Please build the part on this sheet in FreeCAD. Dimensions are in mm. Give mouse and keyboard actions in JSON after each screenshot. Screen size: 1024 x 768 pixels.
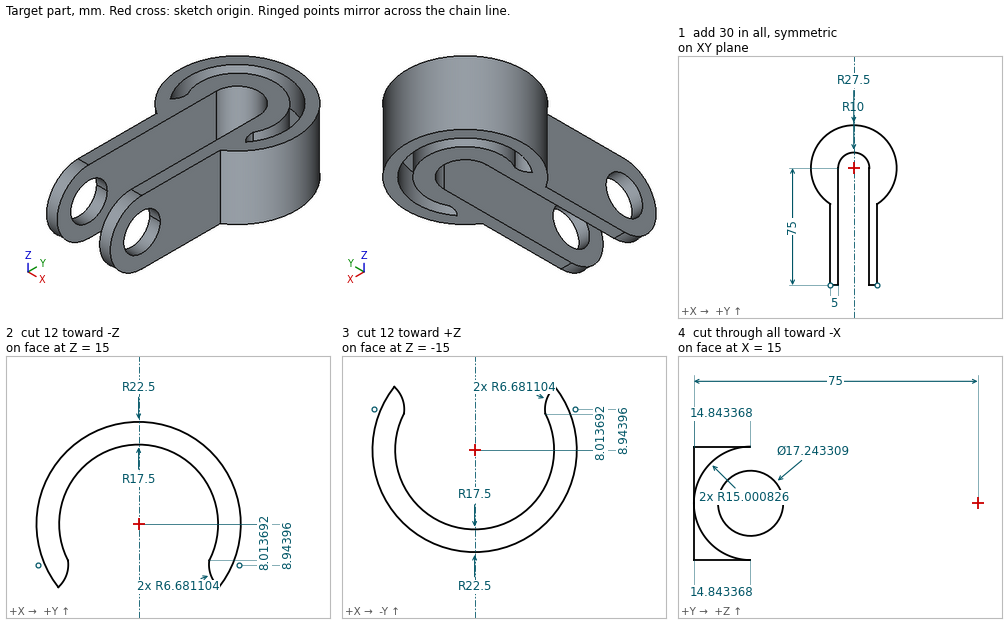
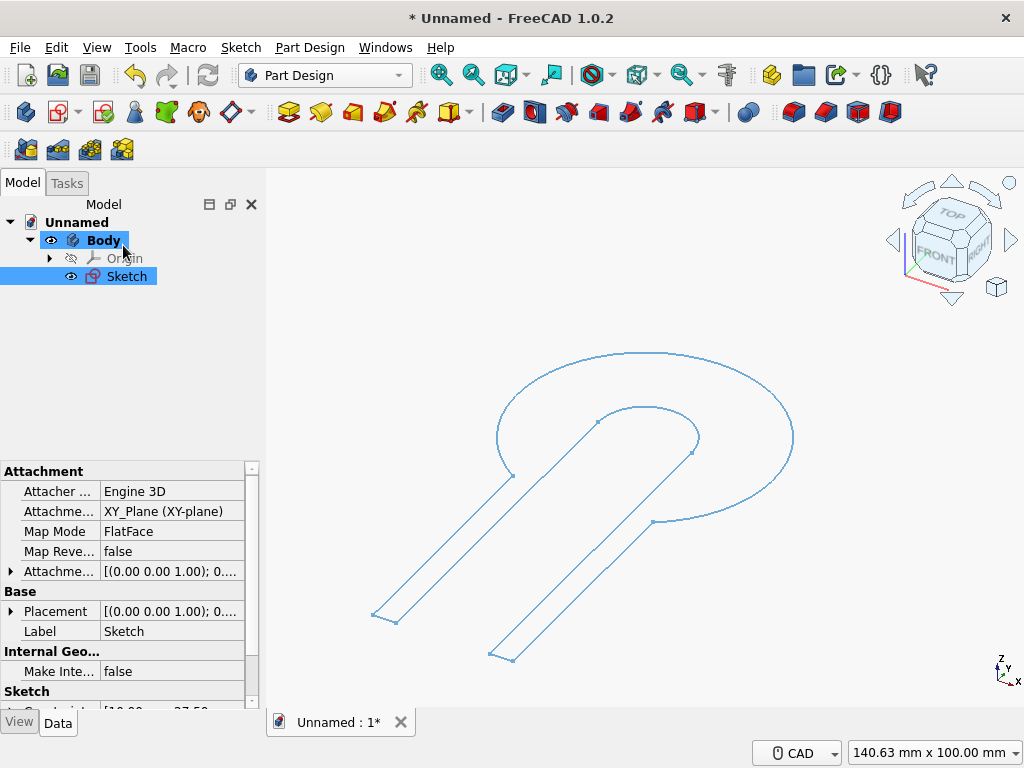
{"action": "left_click", "coordinate": [290, 112]}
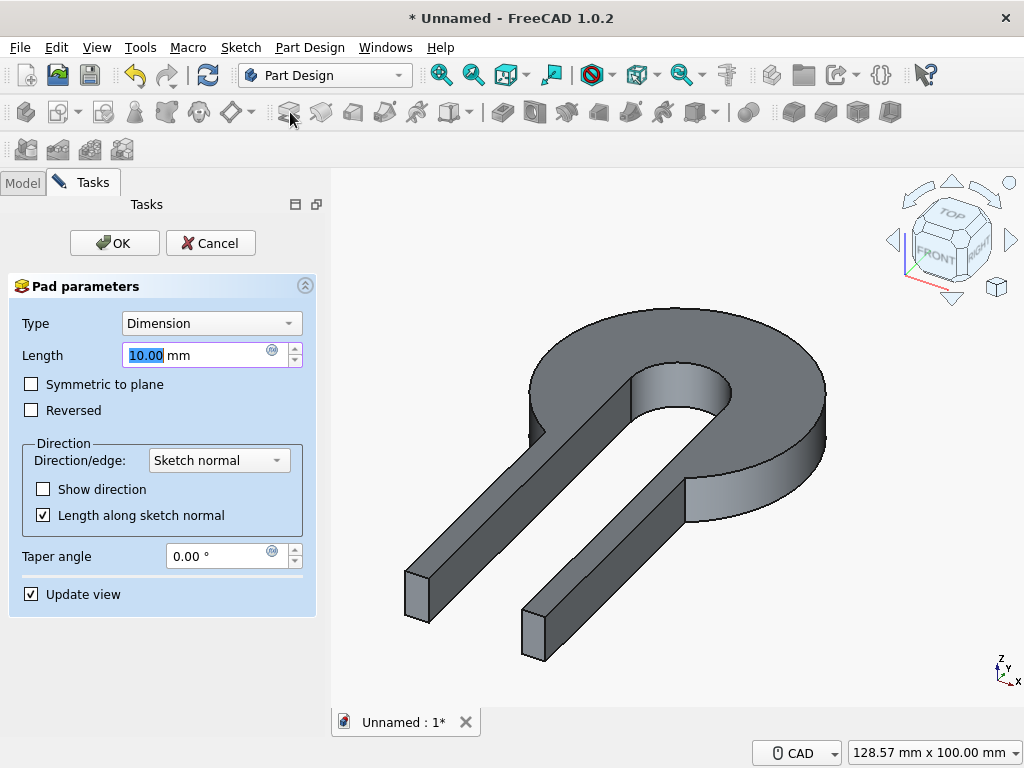
{"action": "type", "text": "30"}
{"action": "key", "text": "Tab"}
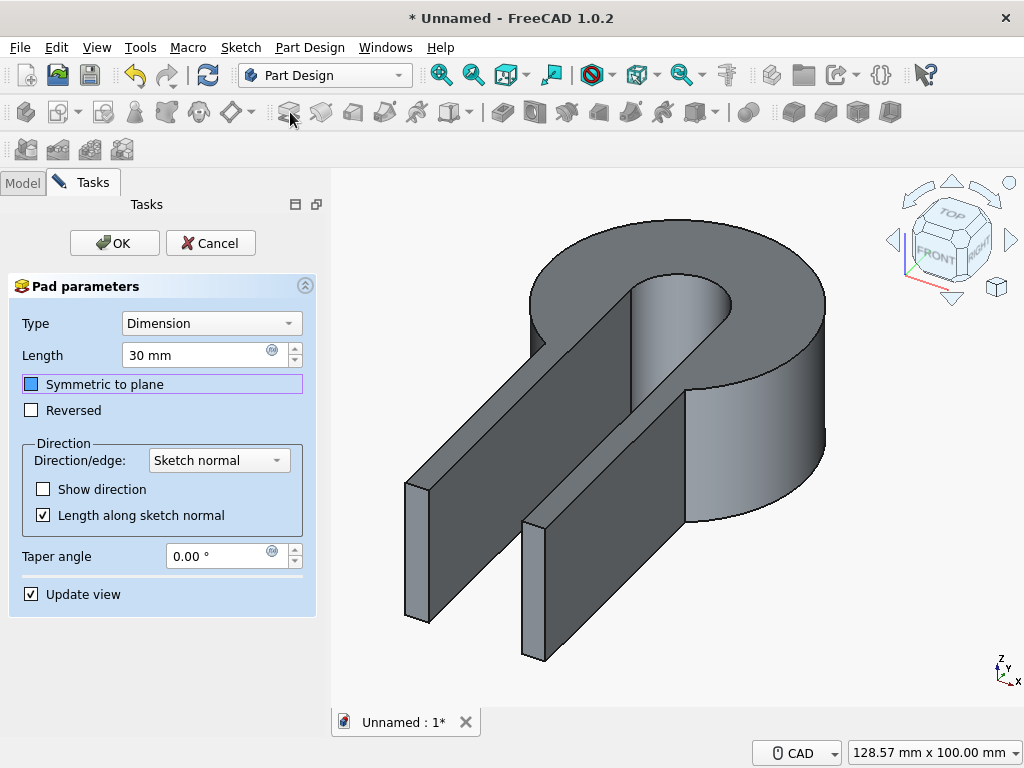
{"action": "left_click", "coordinate": [30, 384]}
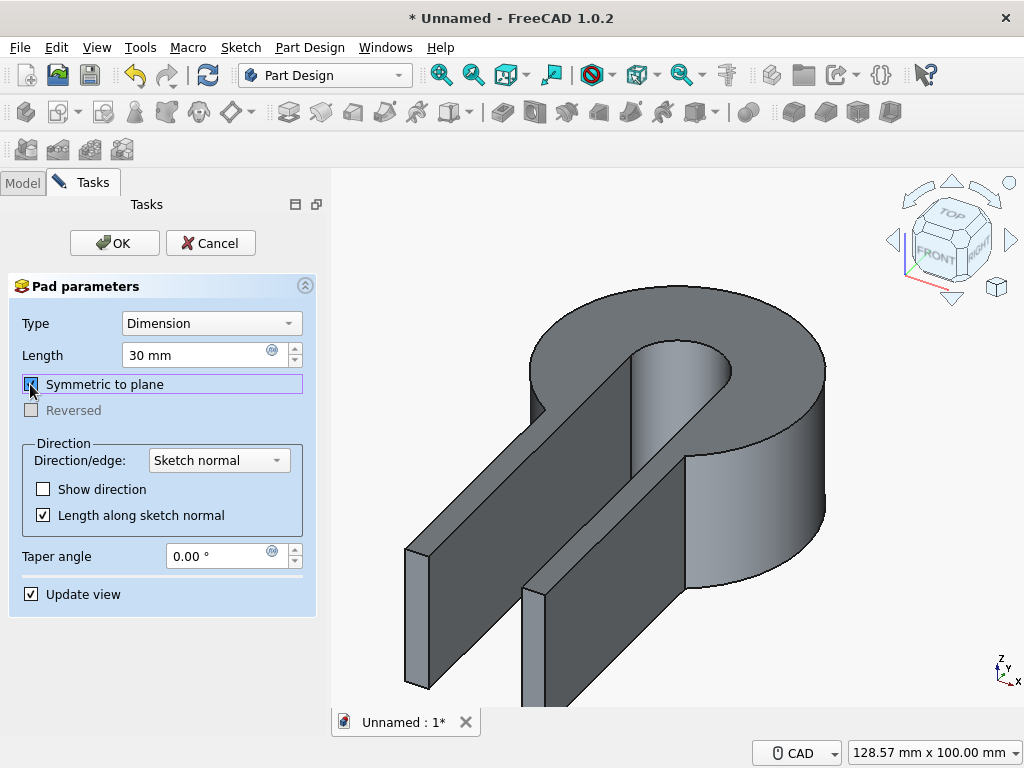
{"action": "left_click", "coordinate": [115, 243]}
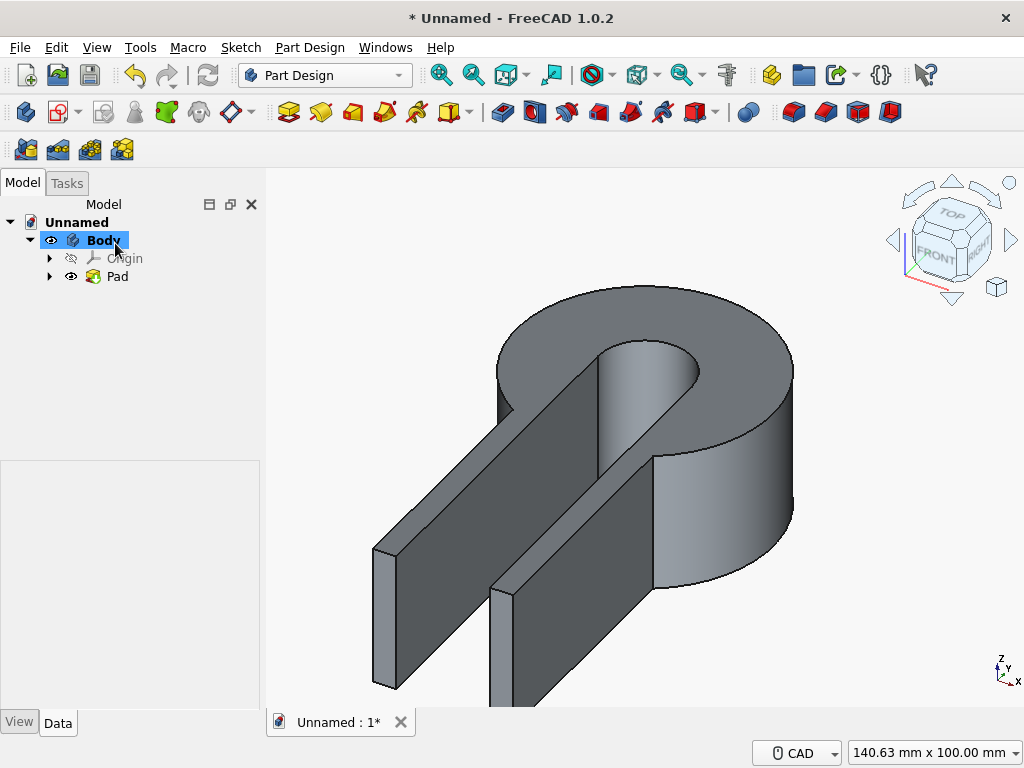
{"action": "key", "text": "v f"}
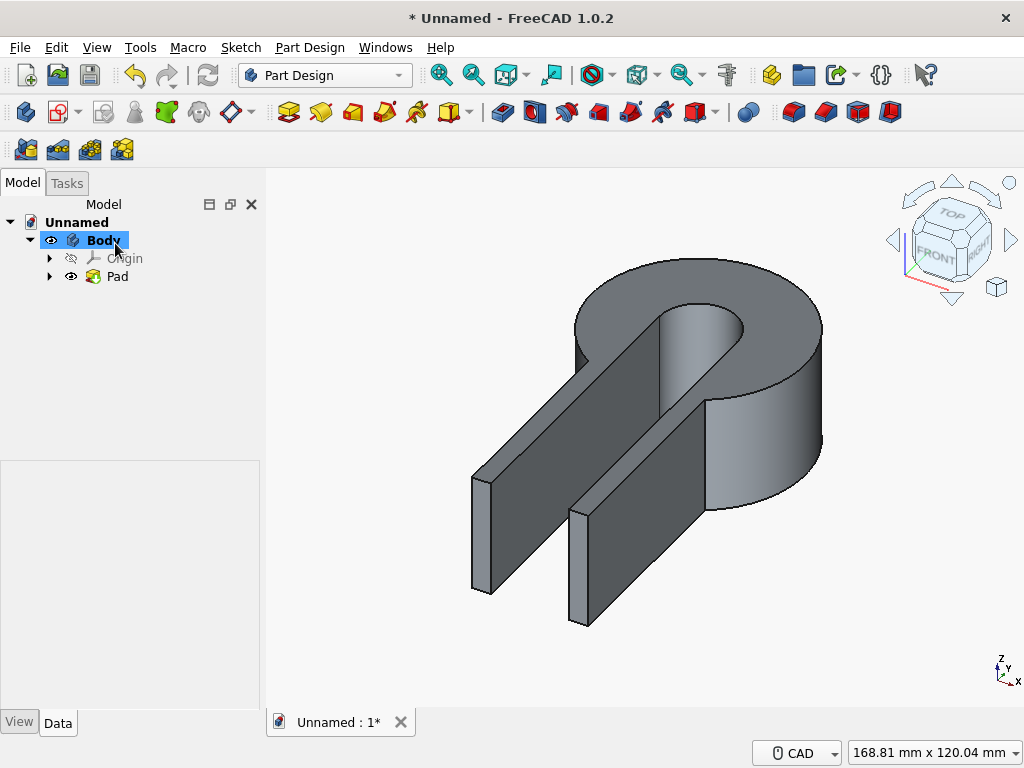
{"action": "left_click", "coordinate": [744, 283]}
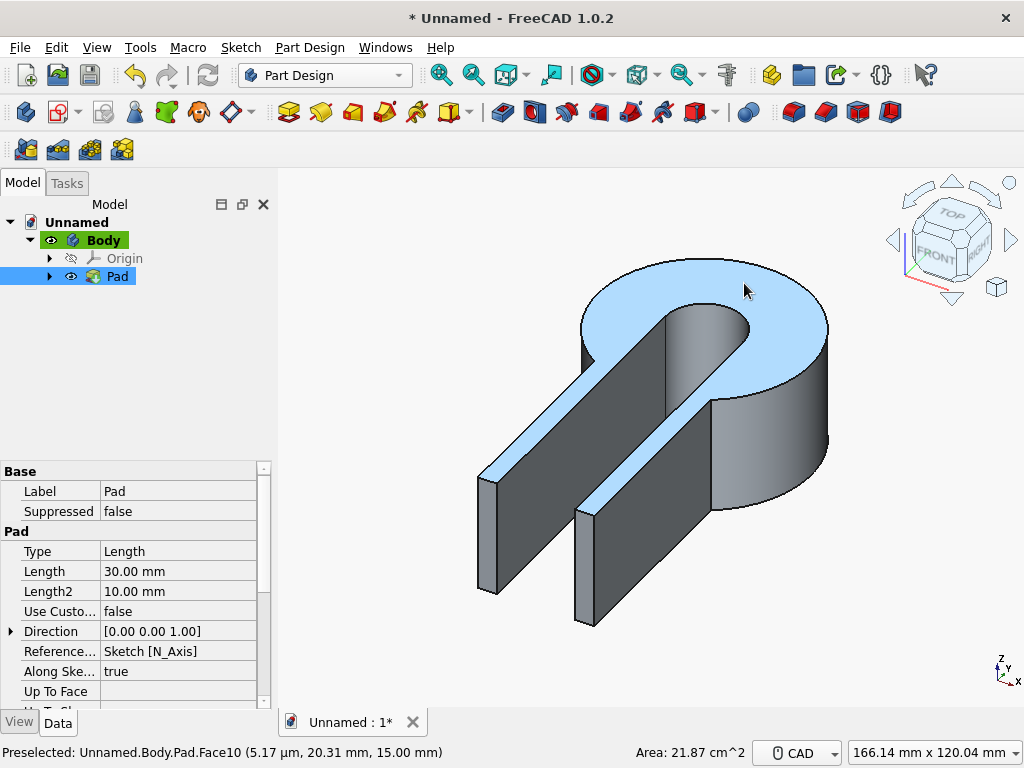
{"action": "left_click", "coordinate": [58, 112]}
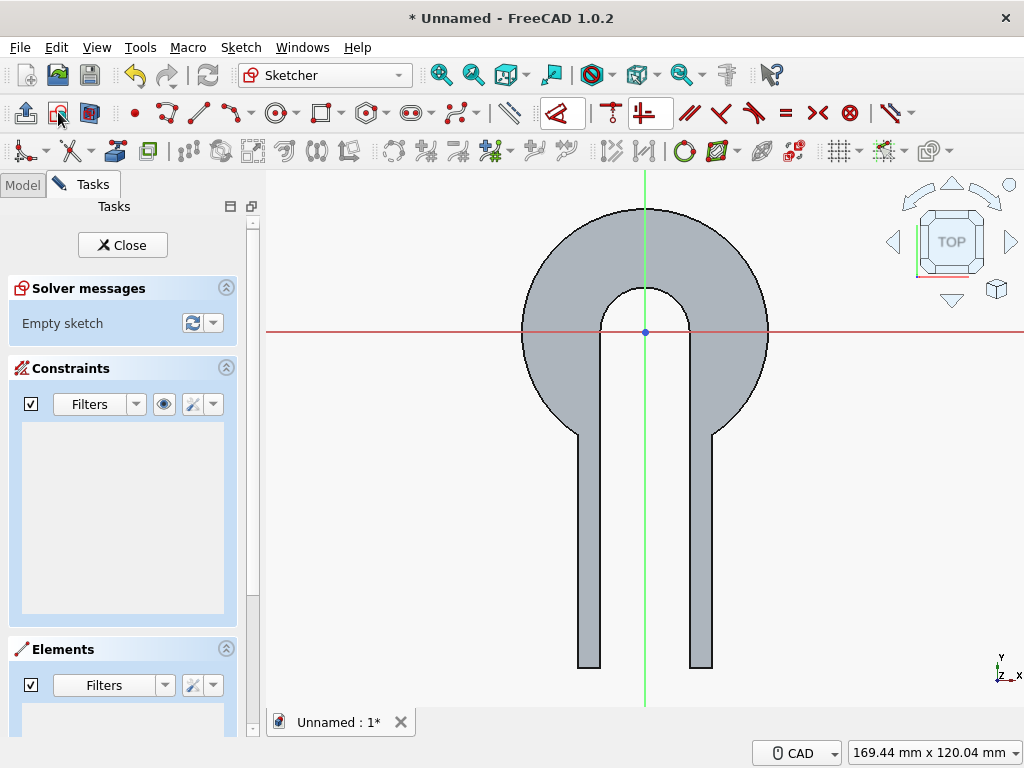
{"action": "scroll", "coordinate": [701, 210], "scroll_direction": "up", "scroll_amount": 4}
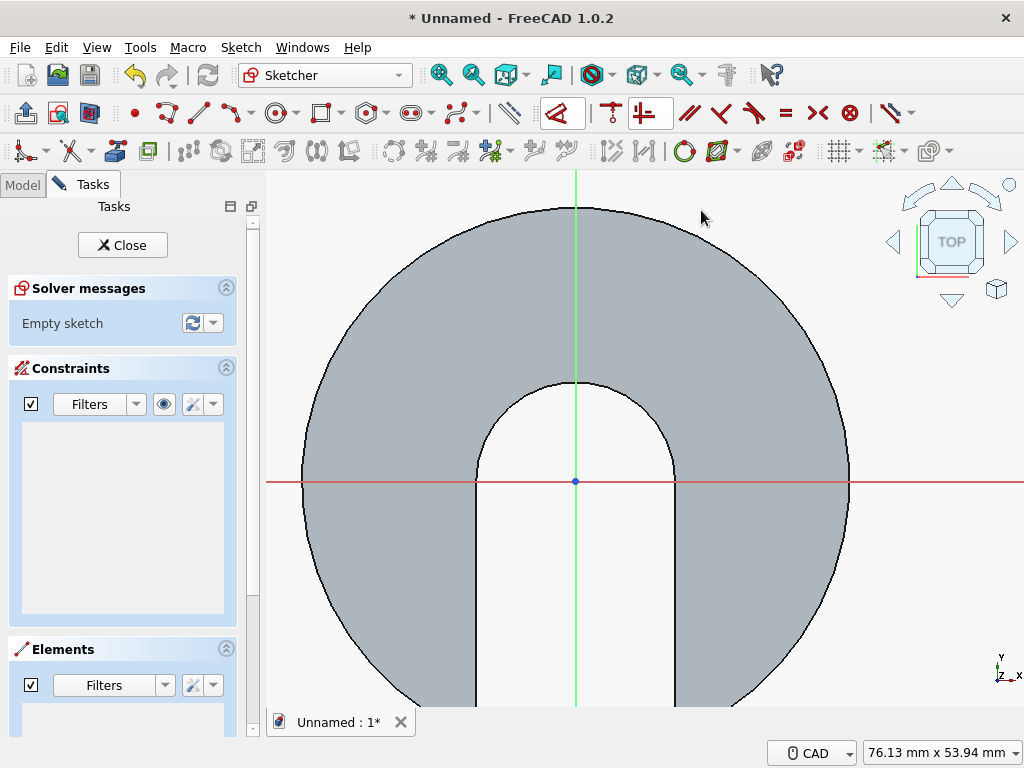
{"action": "key", "text": "g 3 a"}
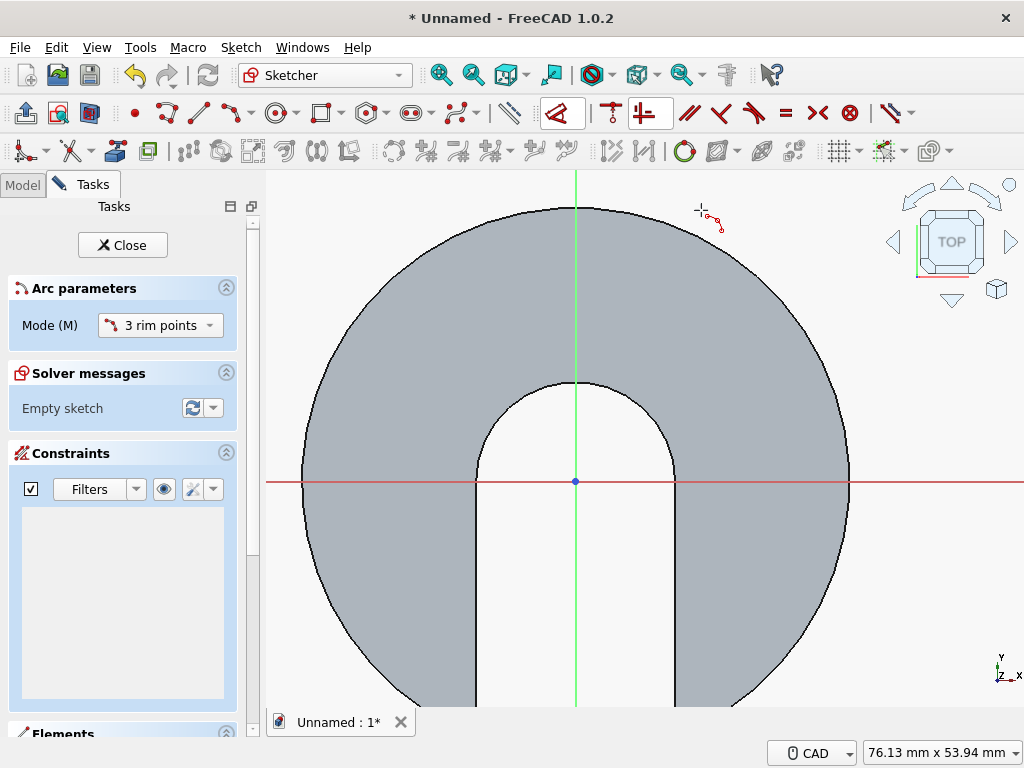
{"action": "left_click", "coordinate": [731, 561]}
{"action": "left_click", "coordinate": [752, 620]}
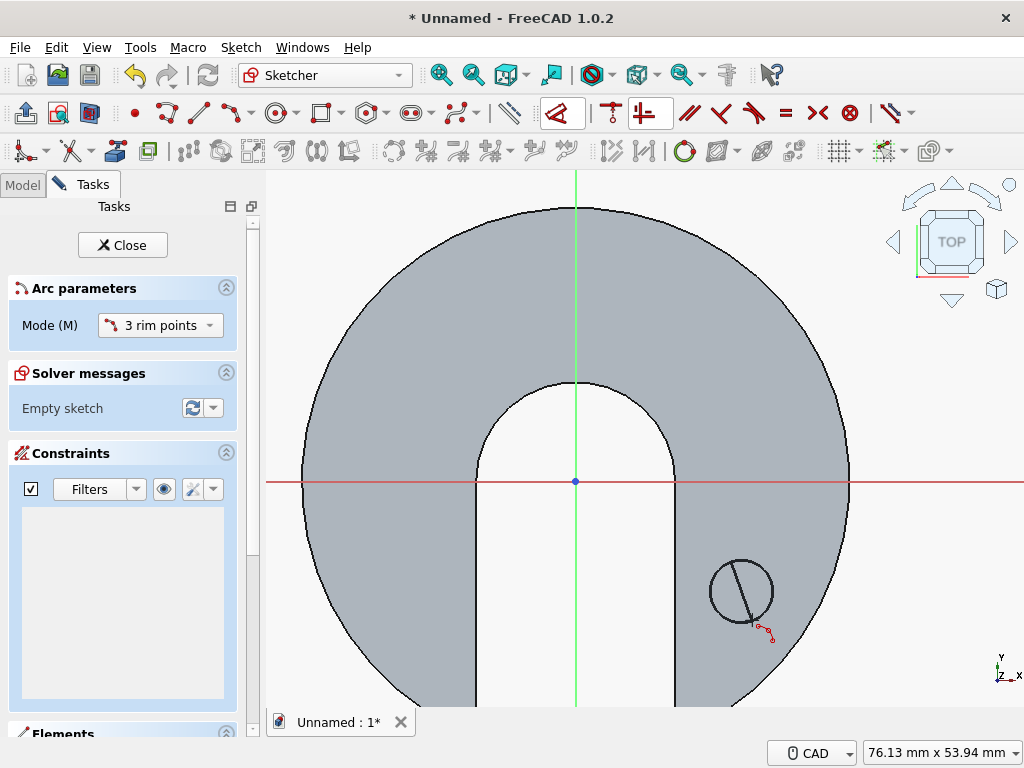
{"action": "scroll", "coordinate": [734, 593], "scroll_direction": "up", "scroll_amount": 4}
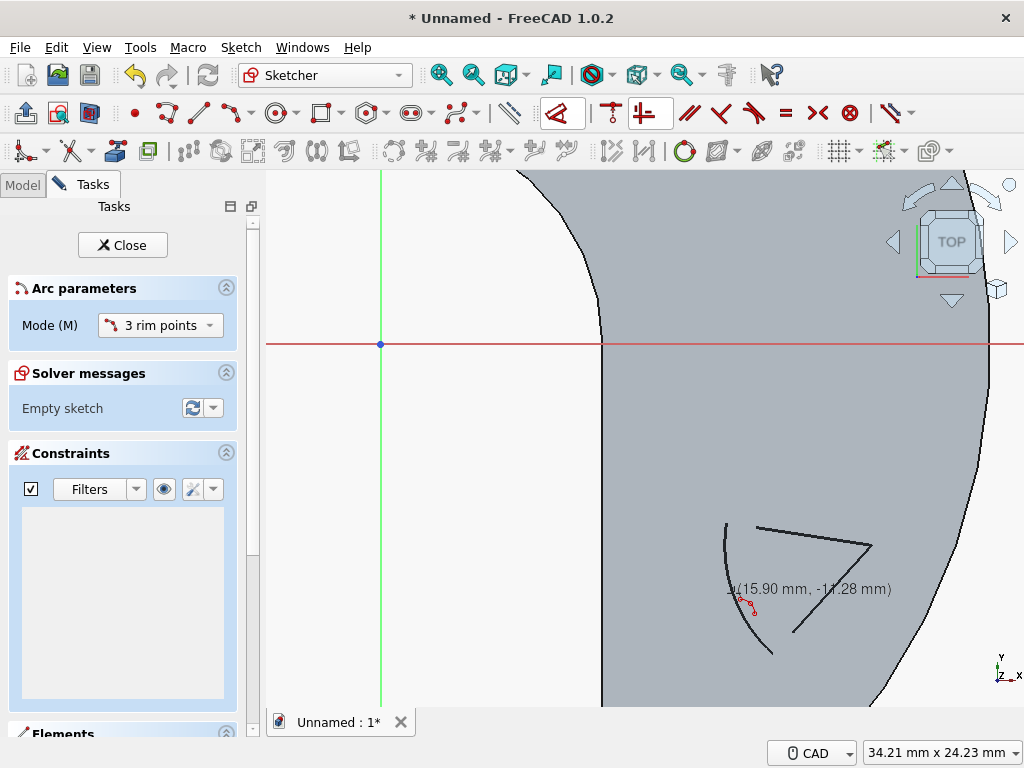
{"action": "left_click", "coordinate": [733, 593]}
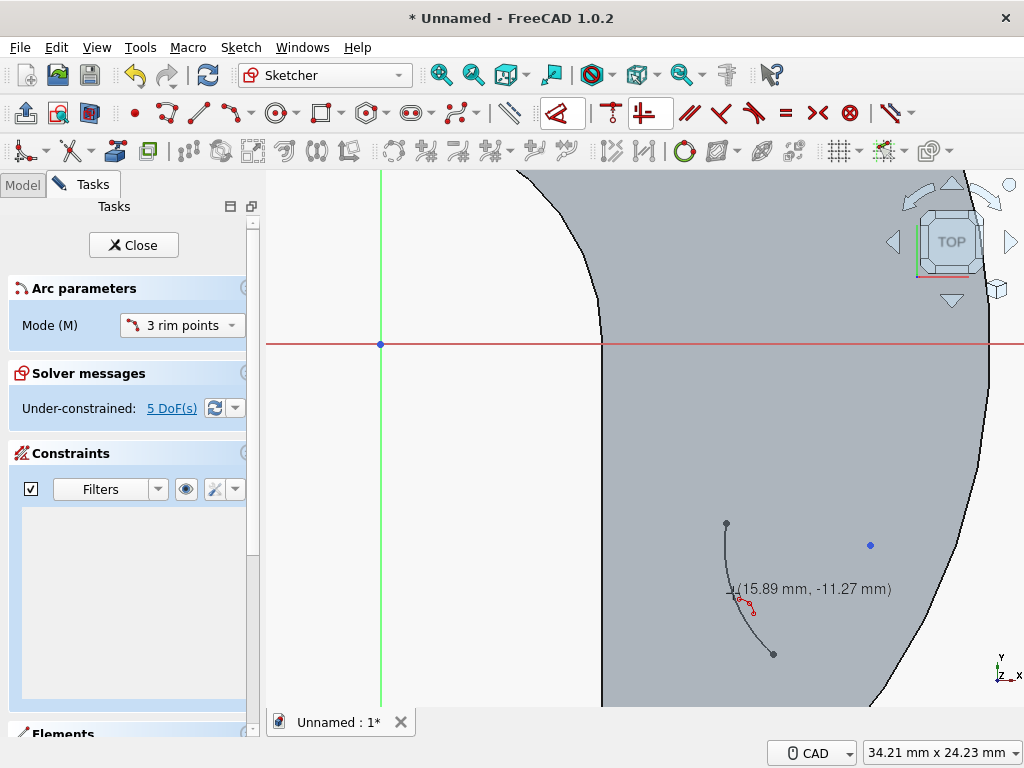
{"action": "left_click", "coordinate": [773, 654]}